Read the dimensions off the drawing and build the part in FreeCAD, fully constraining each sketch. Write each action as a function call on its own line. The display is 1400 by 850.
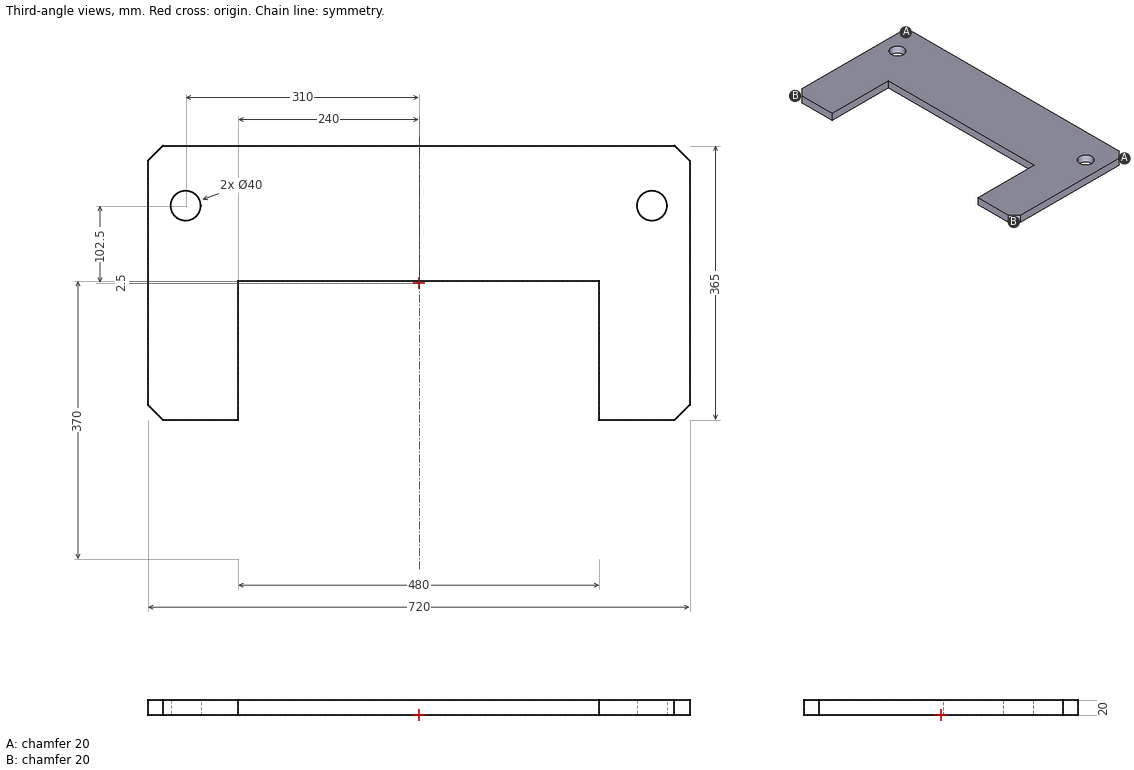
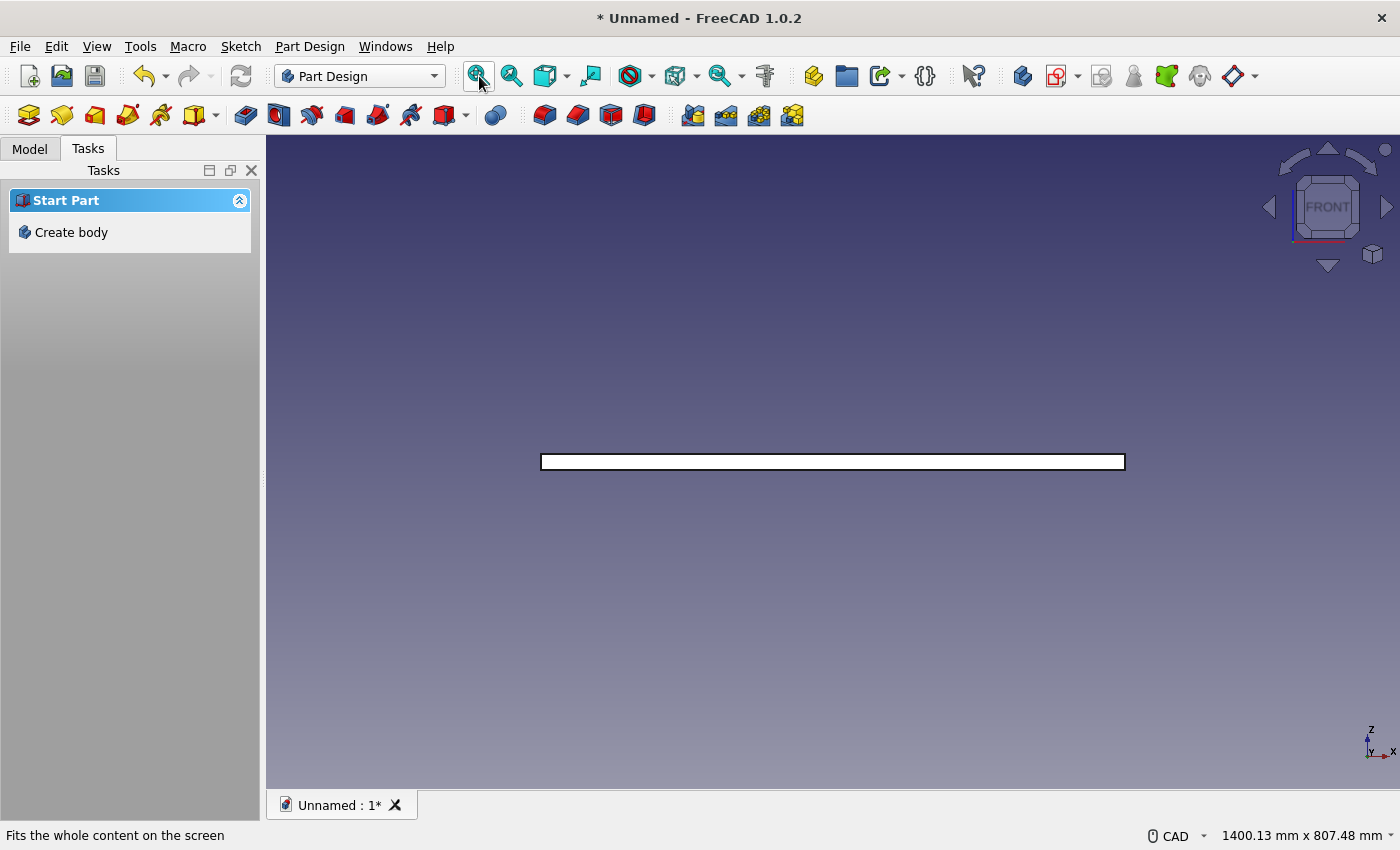
scroll(541, 461, up, 5)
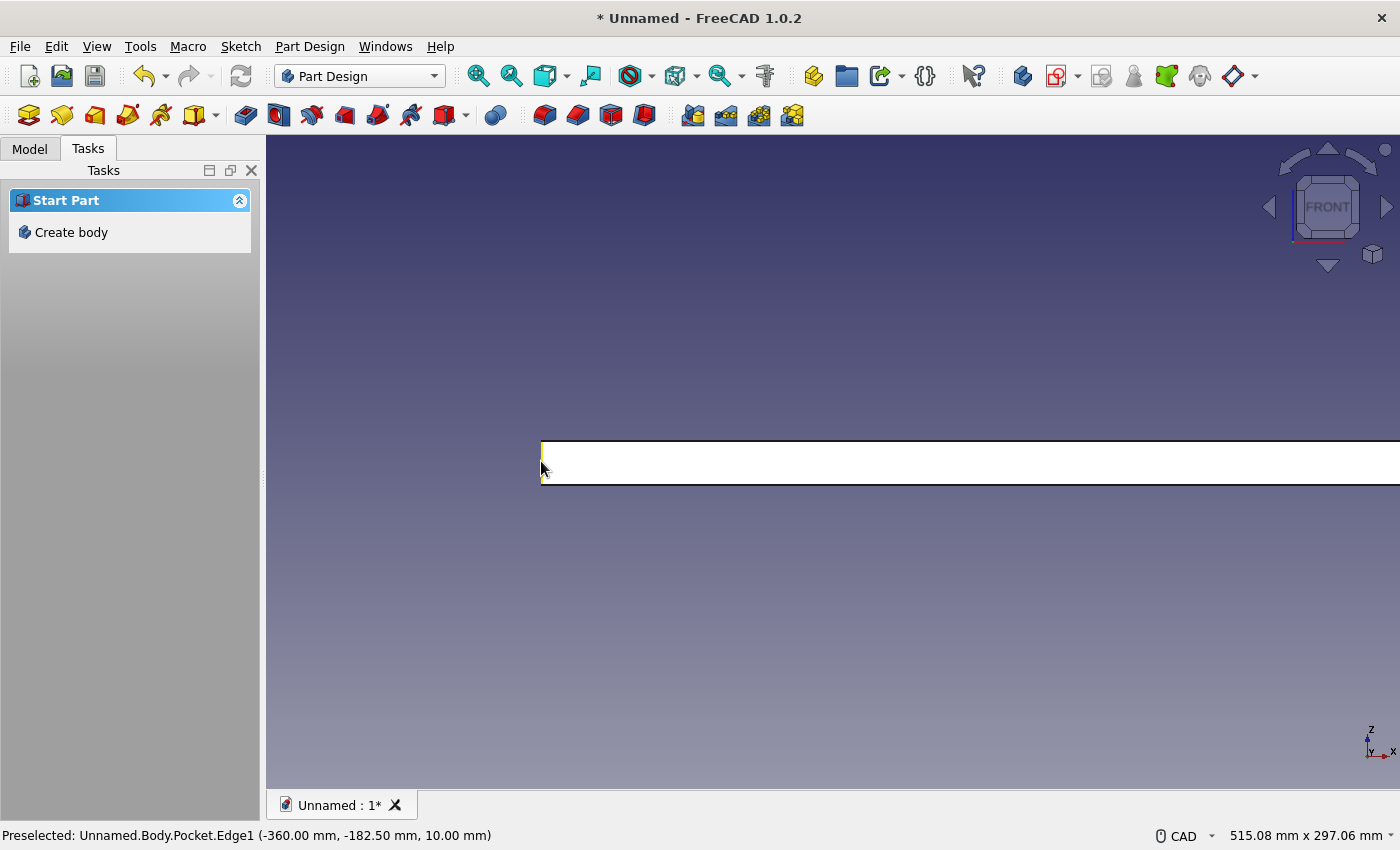
key(v)
key(f)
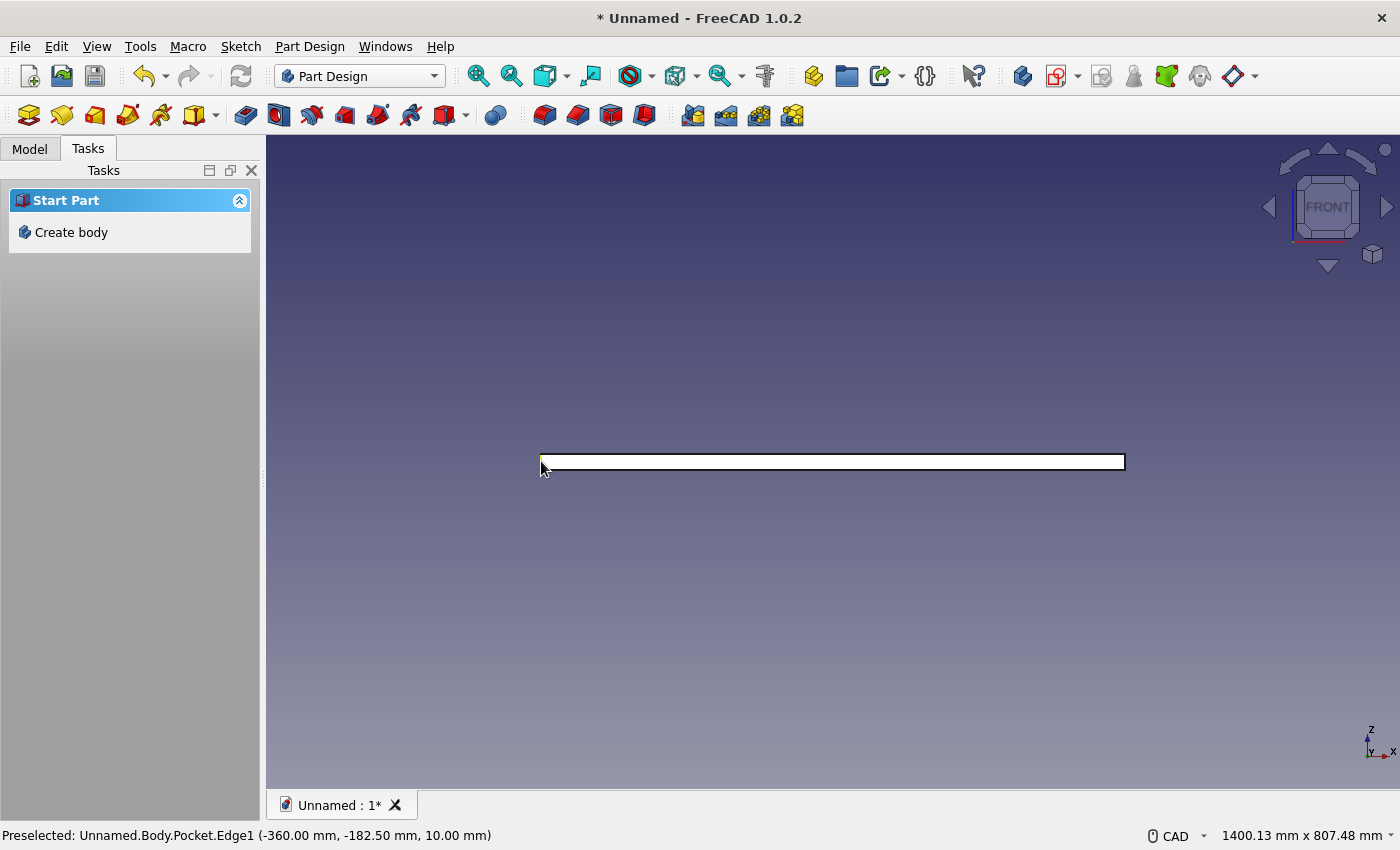
key(3)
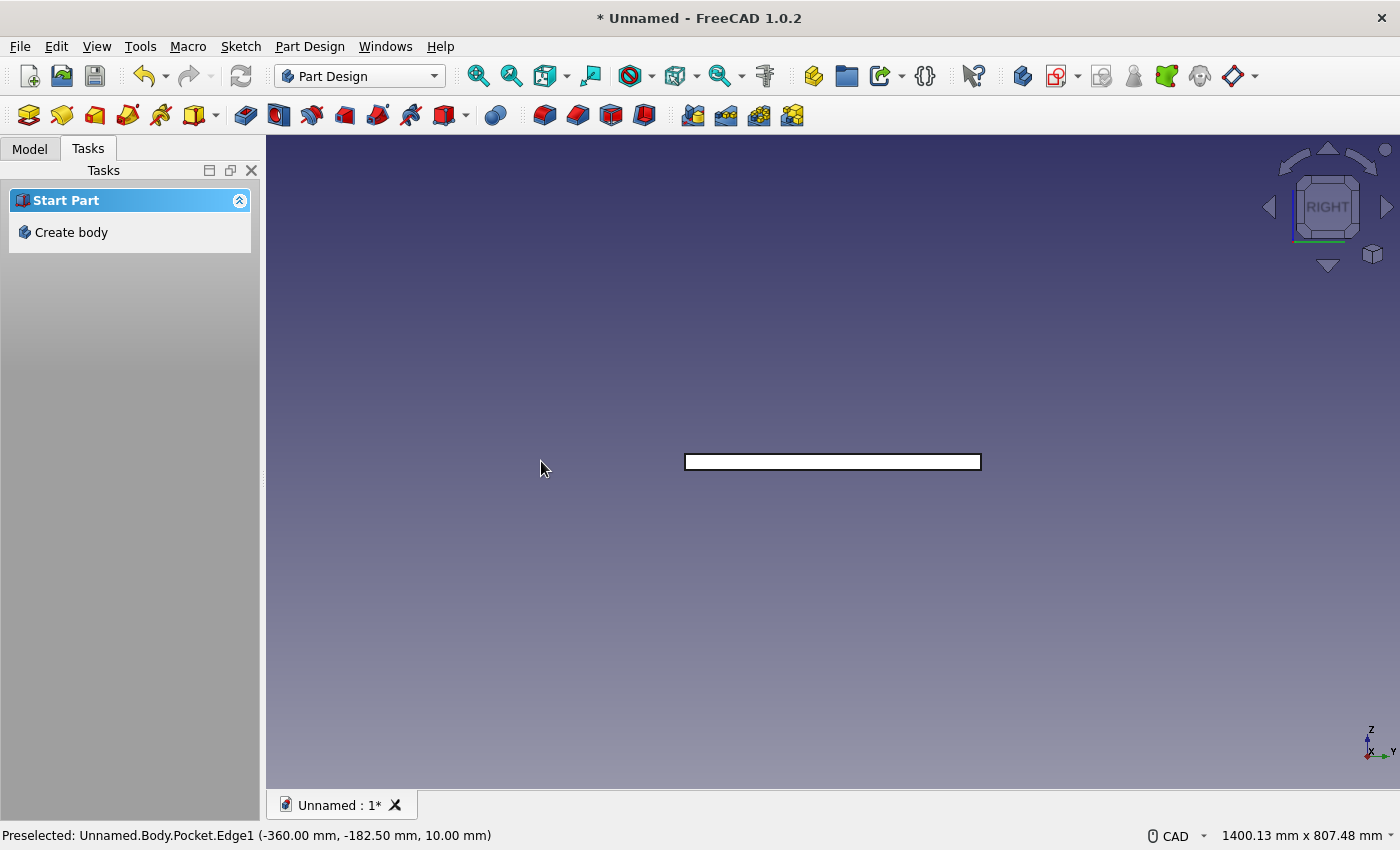
click(479, 76)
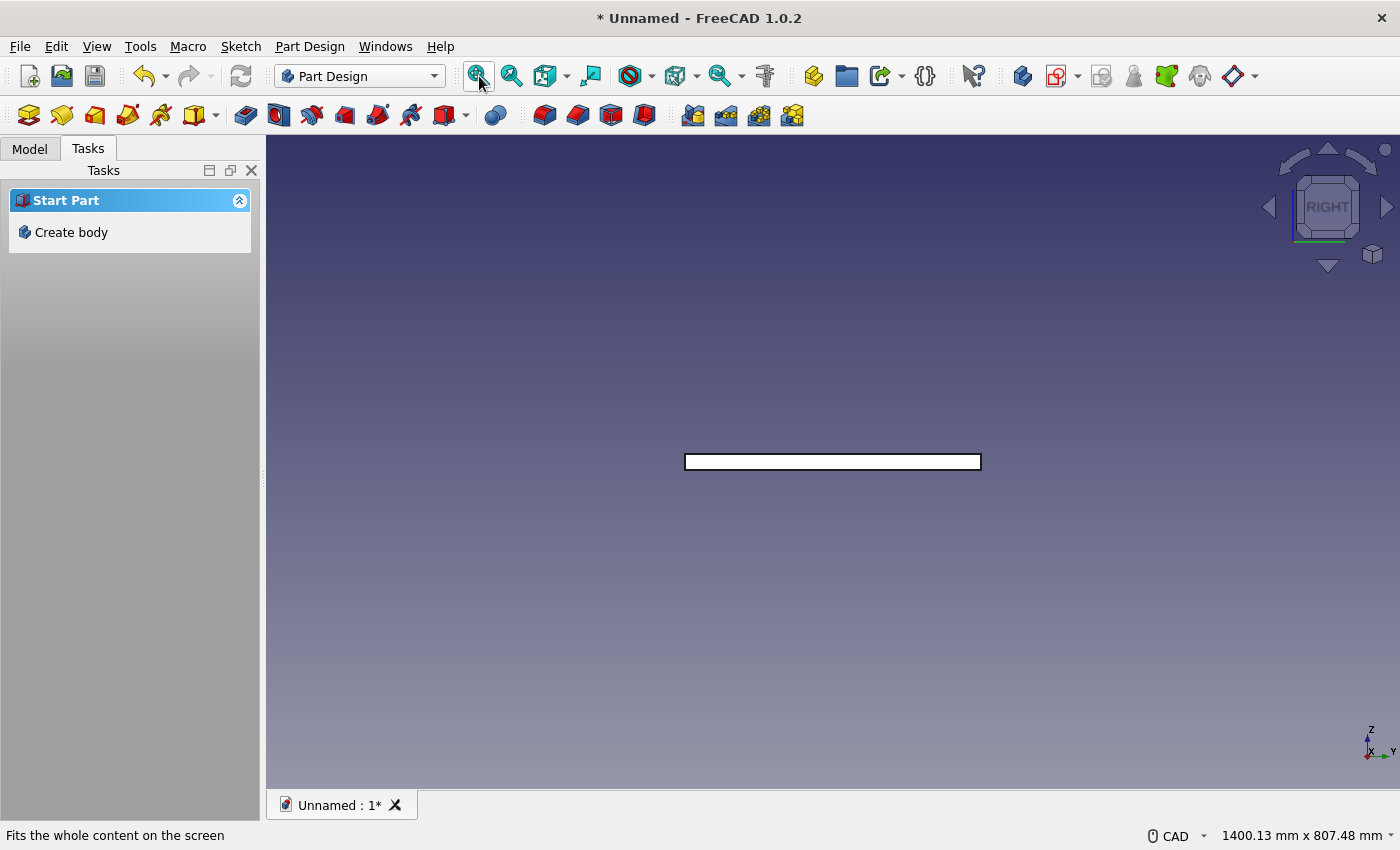
click(981, 461)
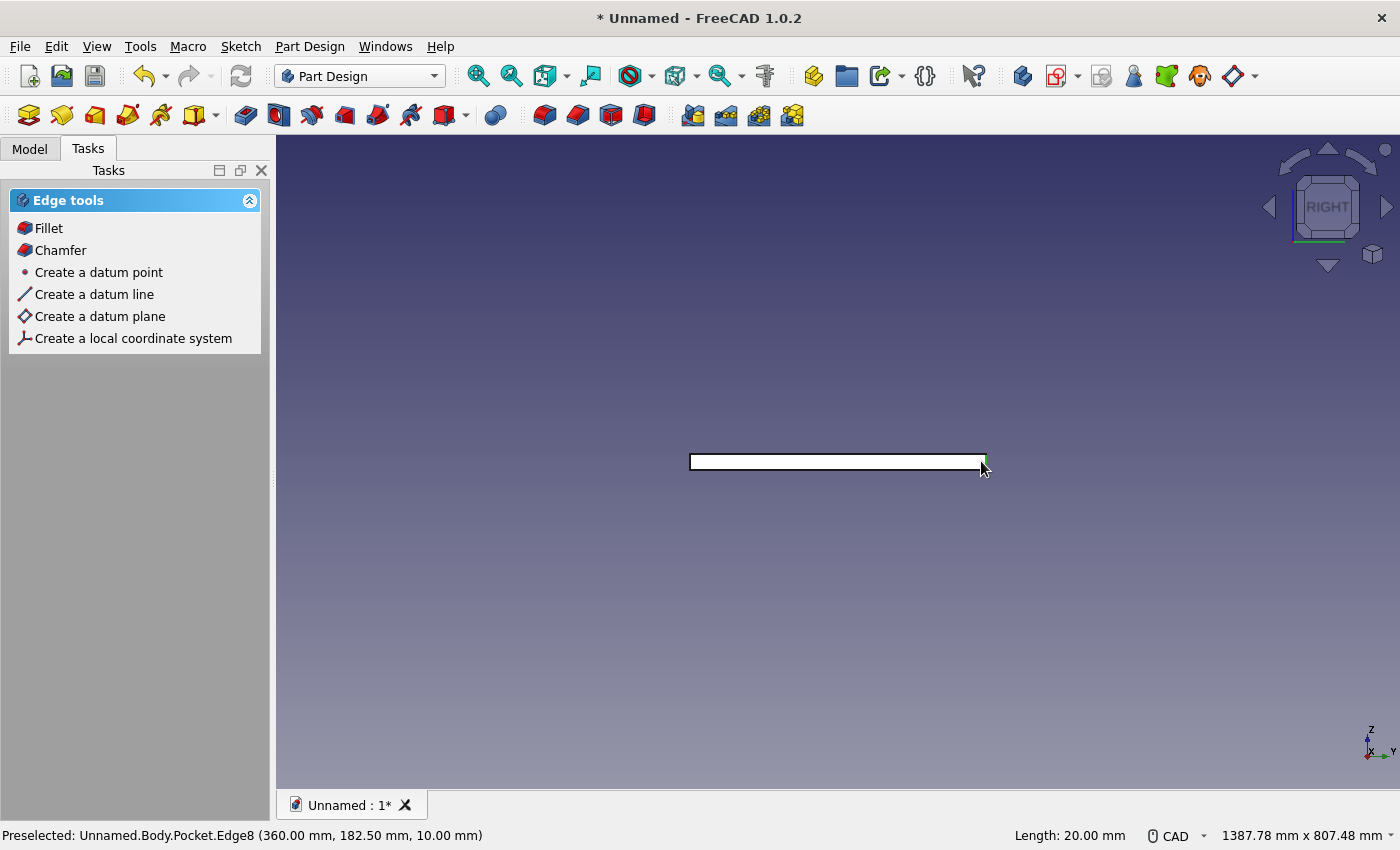
scroll(986, 461, up, 5)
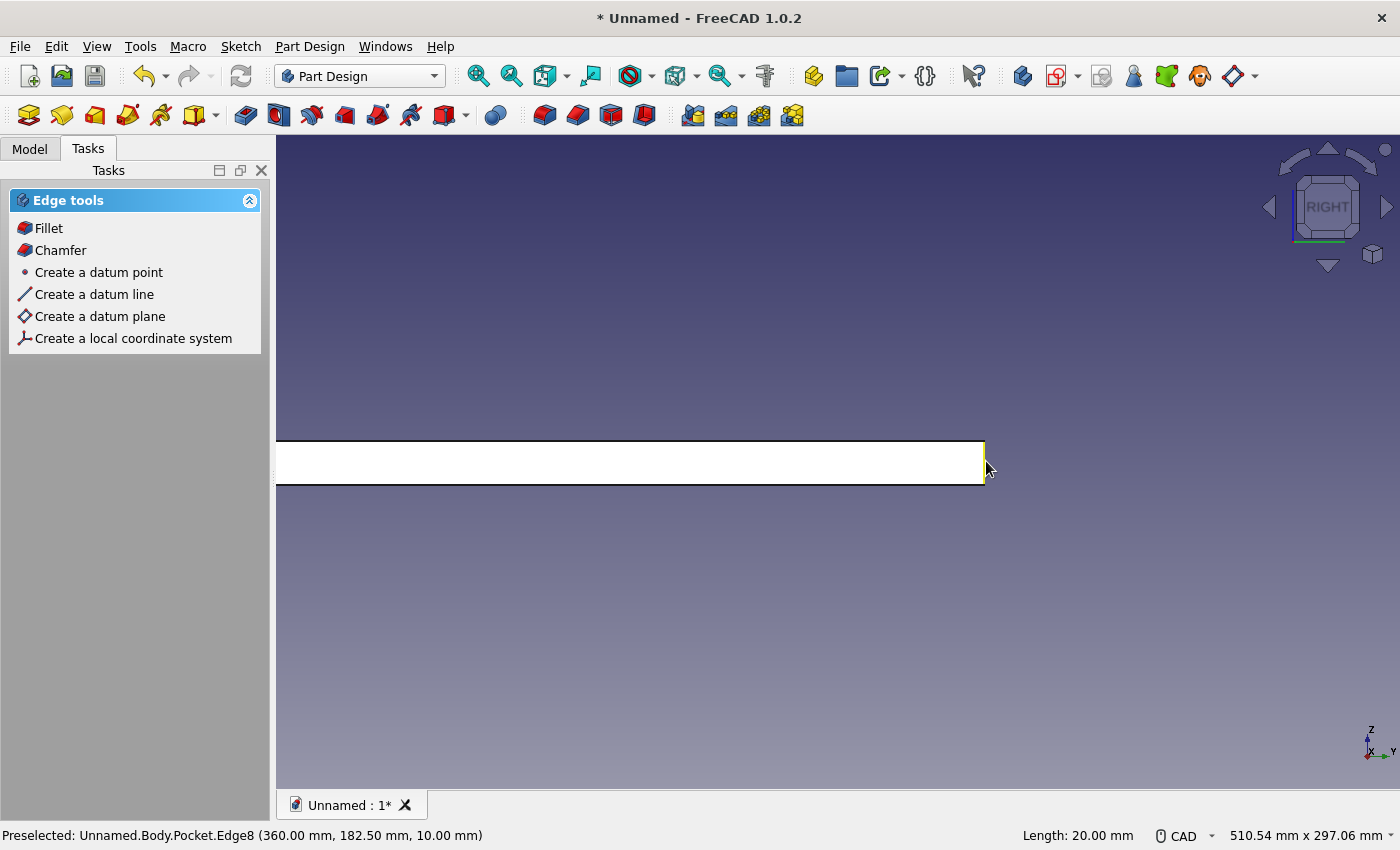
click(479, 76)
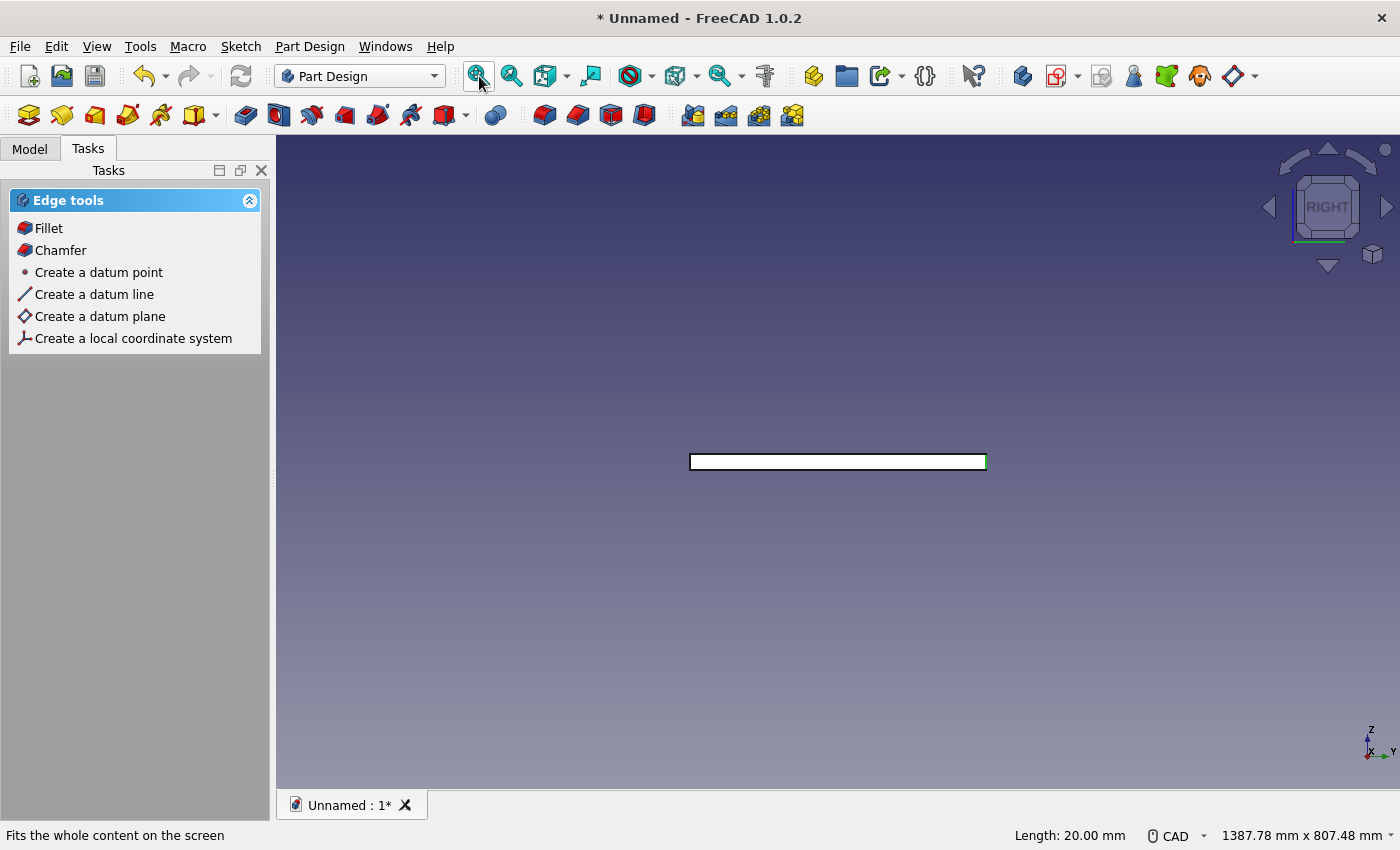
key(5)